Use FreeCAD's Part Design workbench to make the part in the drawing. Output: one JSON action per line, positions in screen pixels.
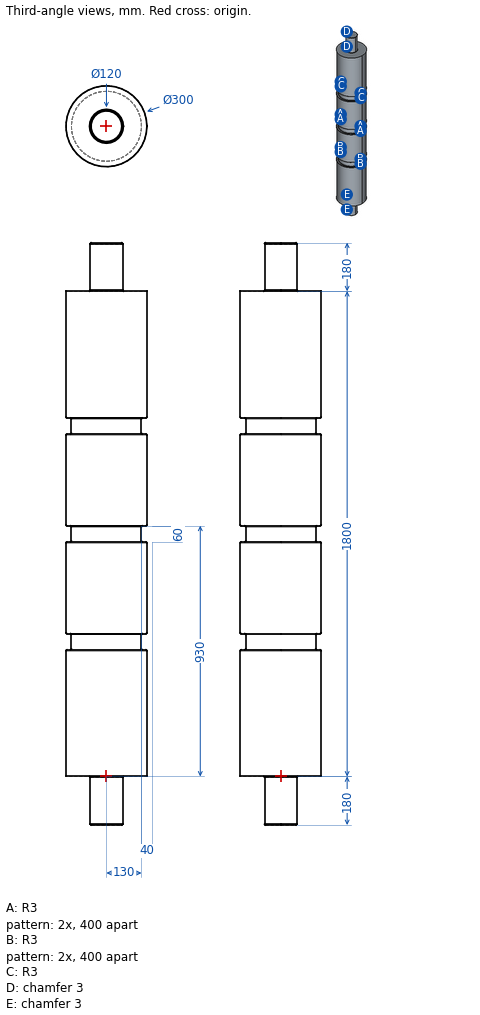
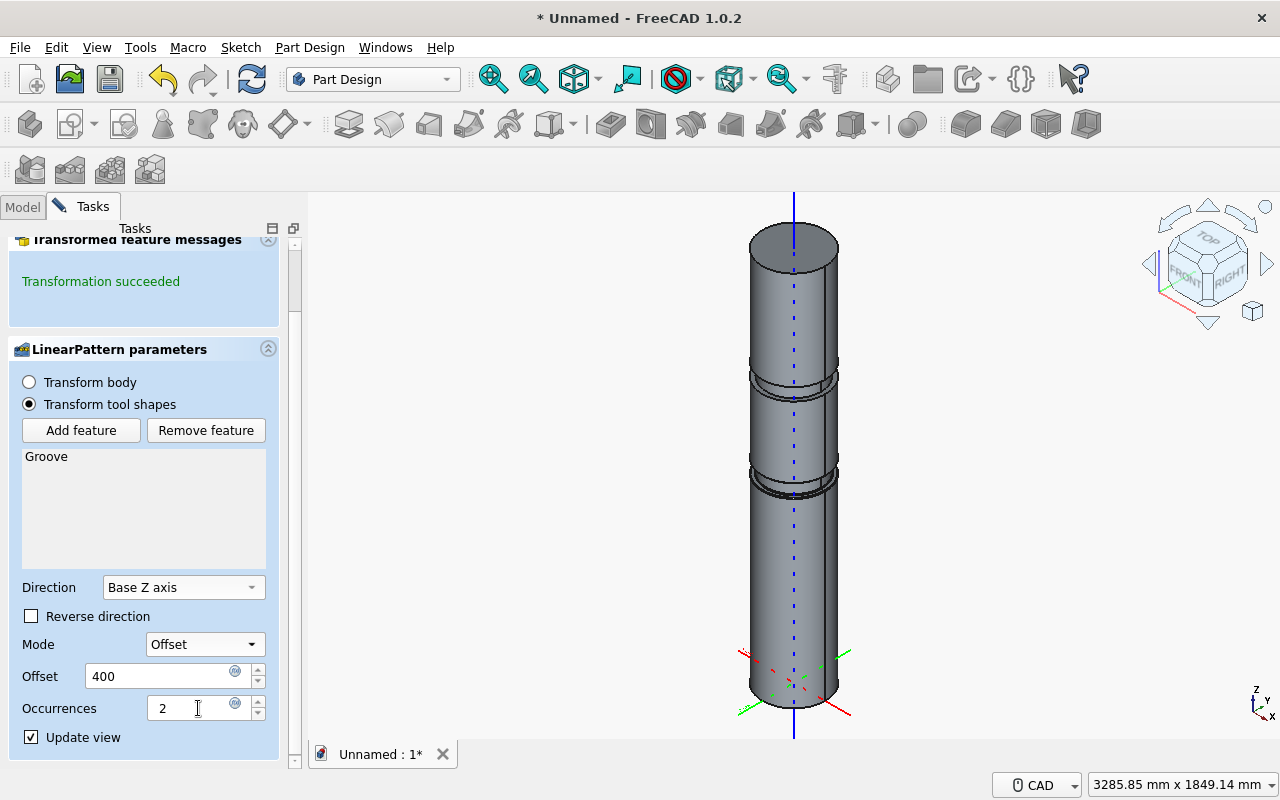
{"action": "left_click", "coordinate": [30, 616]}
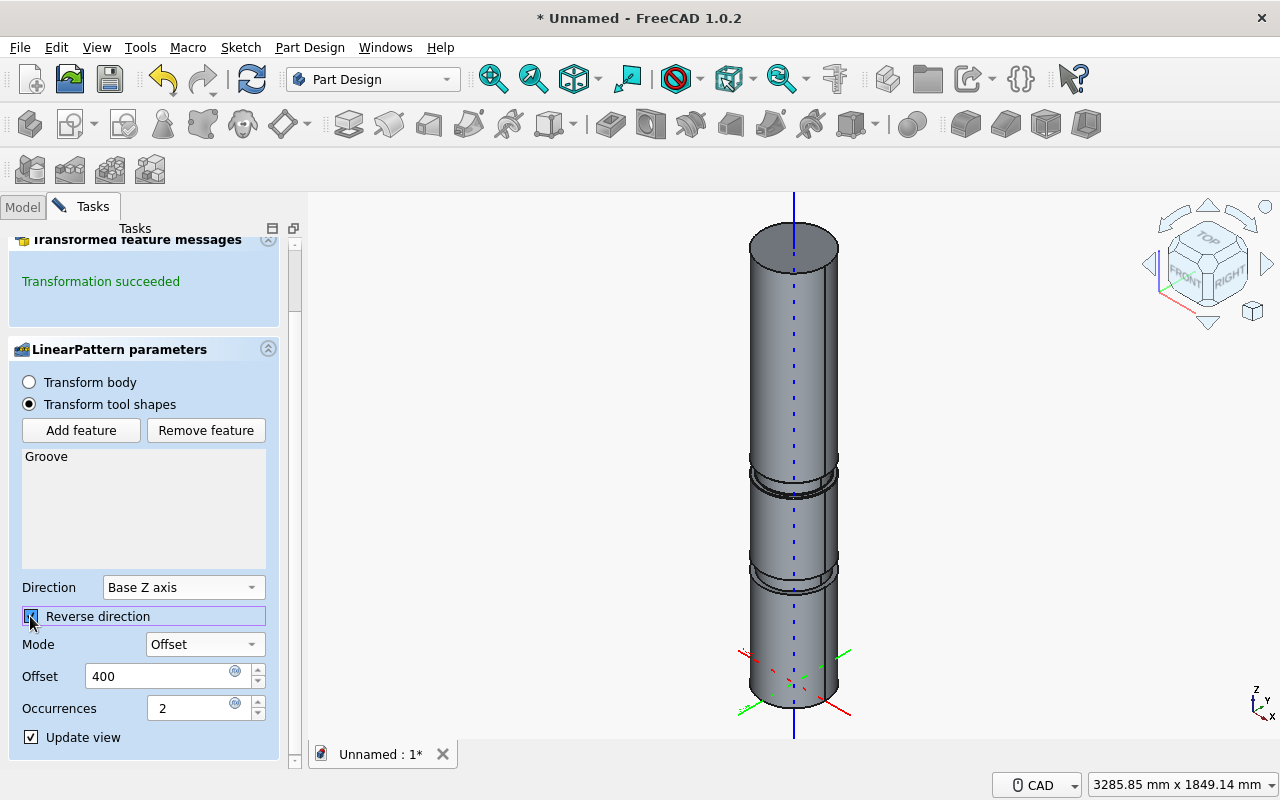
{"action": "scroll", "coordinate": [295, 503], "scroll_direction": "up", "scroll_amount": 2}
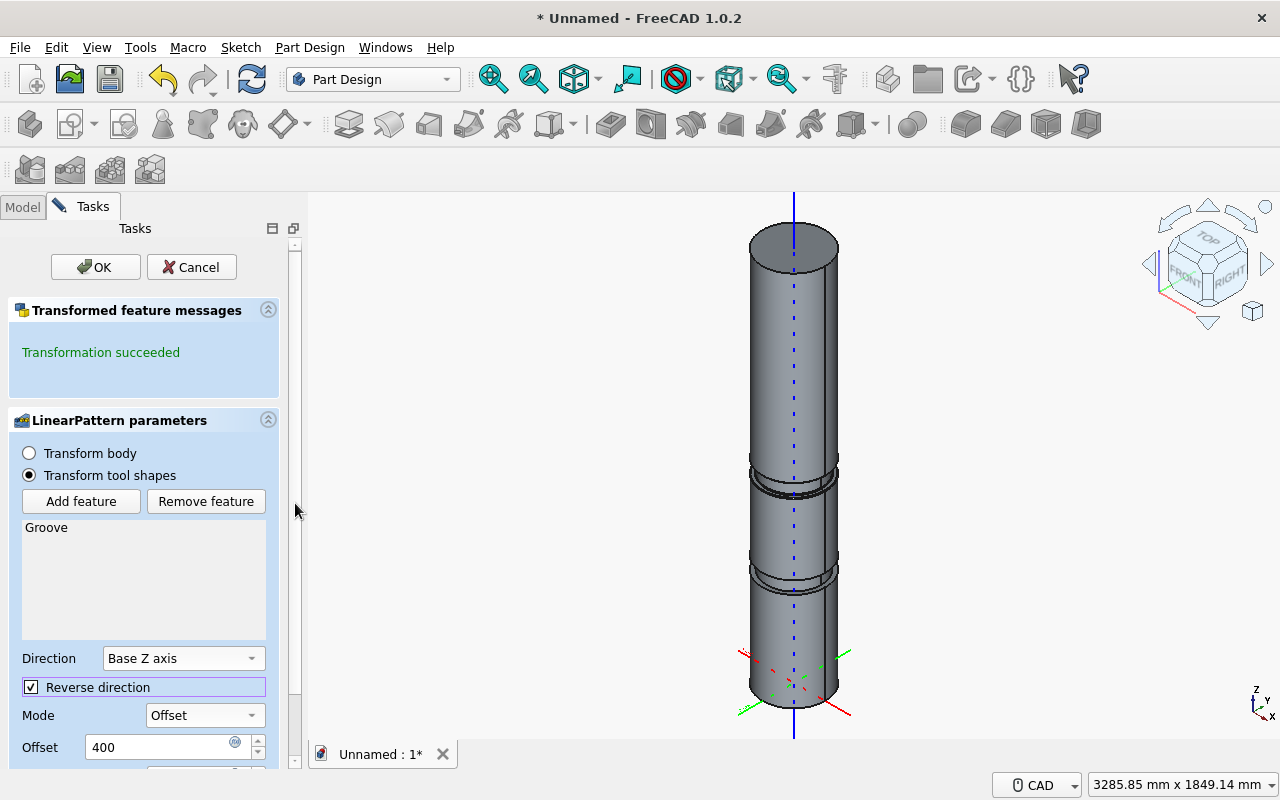
{"action": "left_click", "coordinate": [96, 267]}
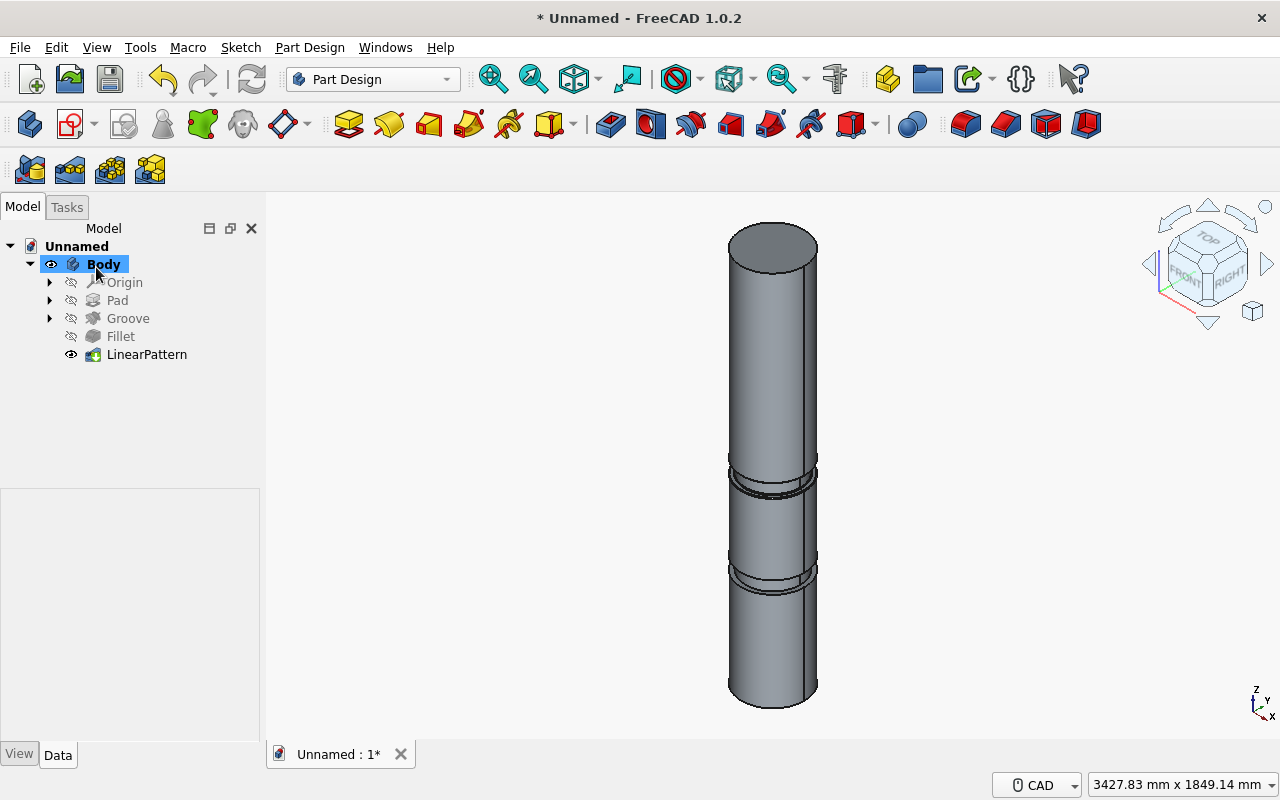
{"action": "left_click", "coordinate": [733, 580]}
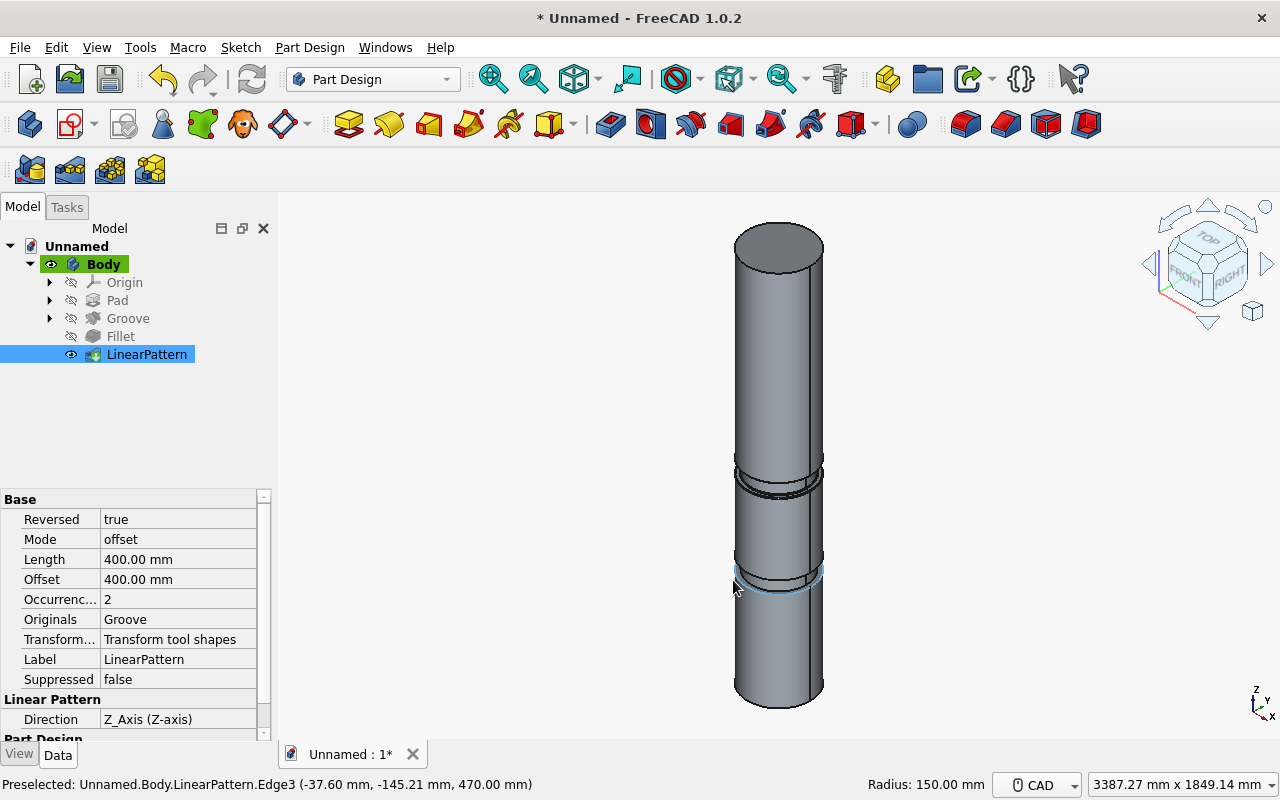
{"action": "key", "text": "2"}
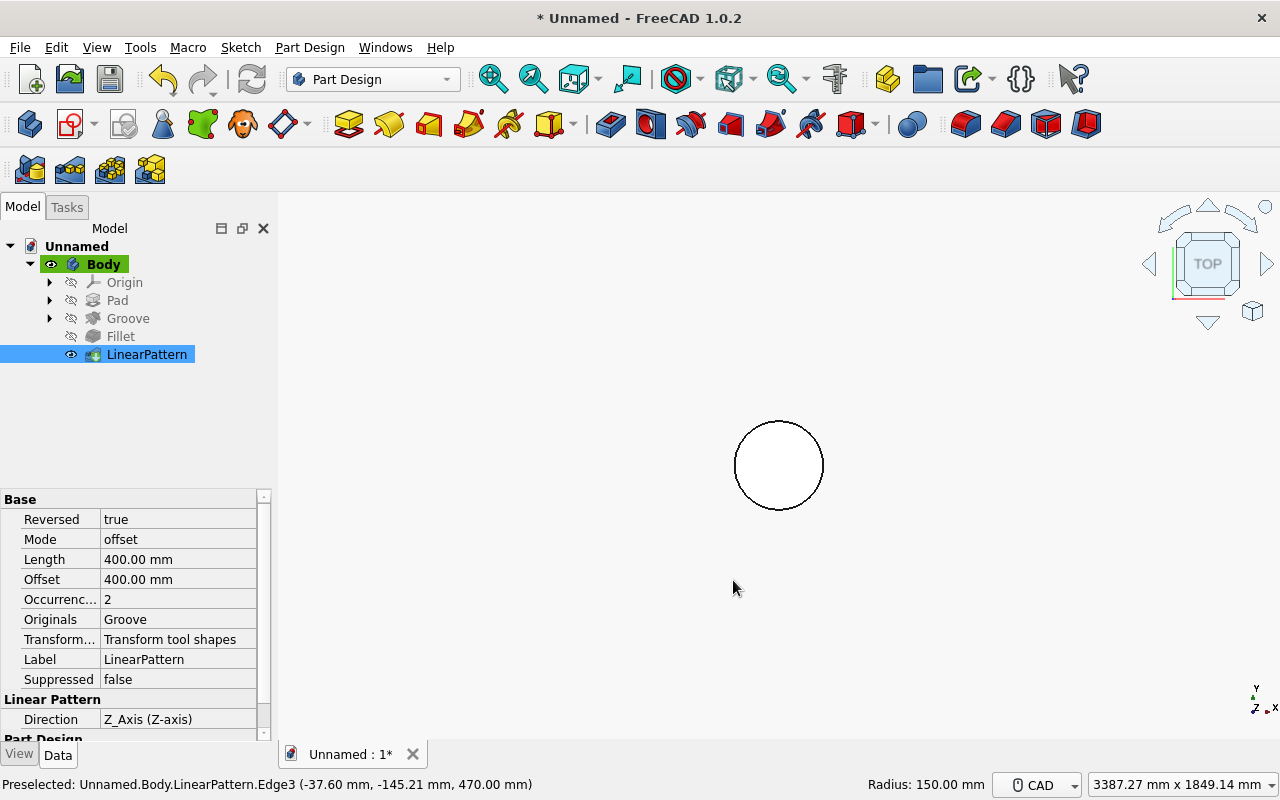
{"action": "key", "text": "v f"}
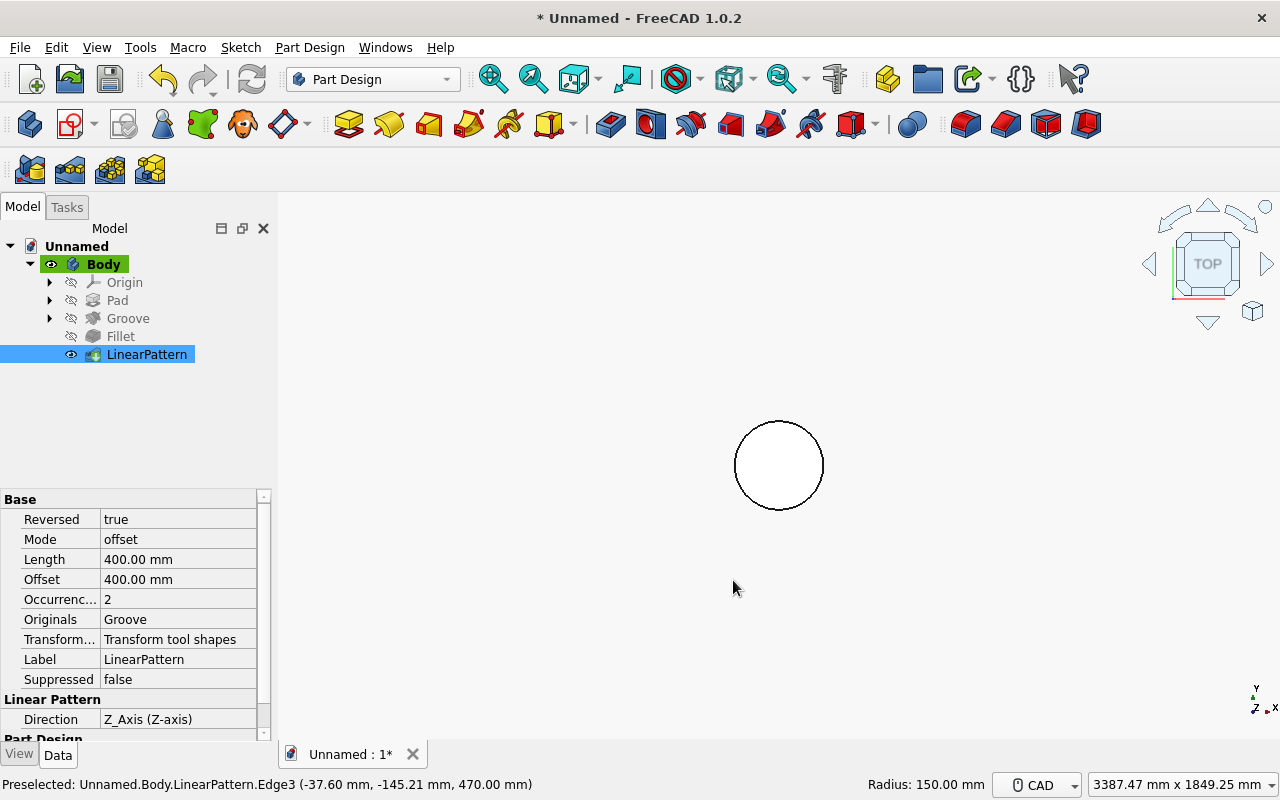
{"action": "key", "text": "0"}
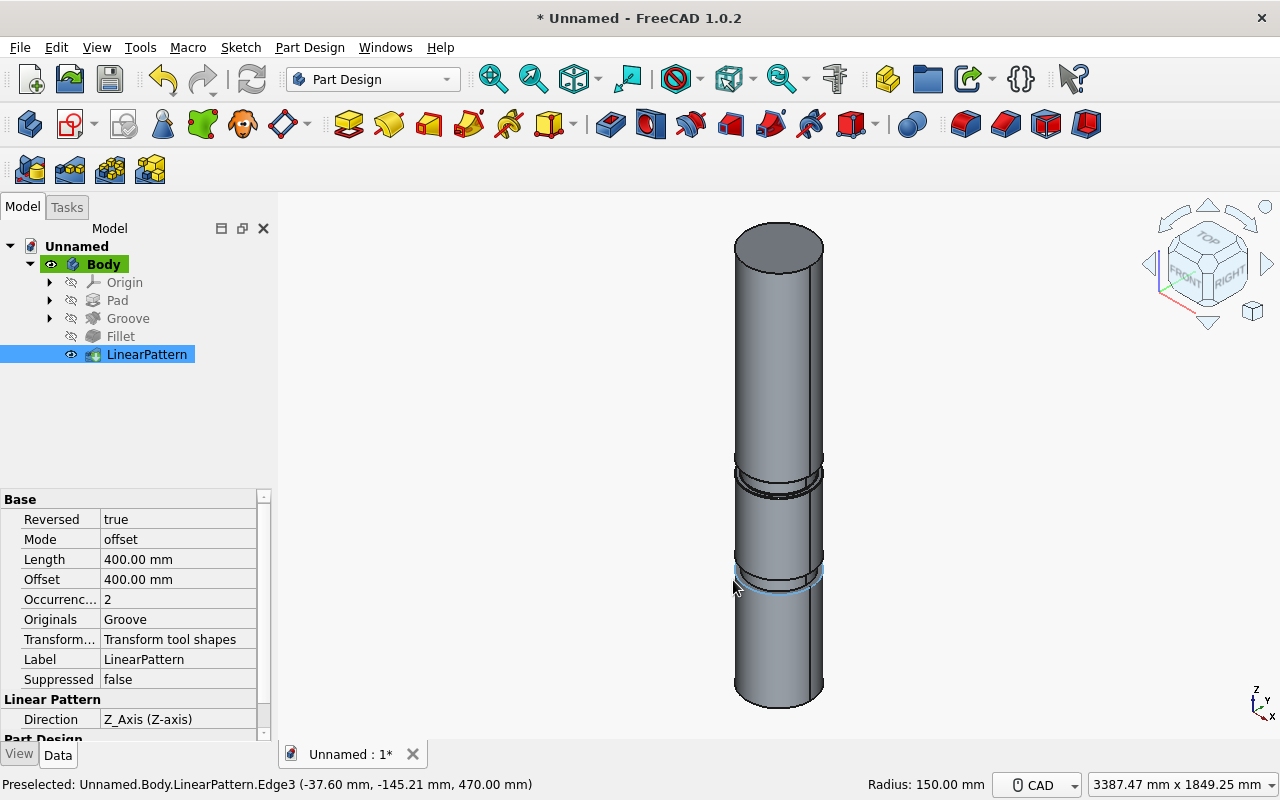
{"action": "key", "text": "1"}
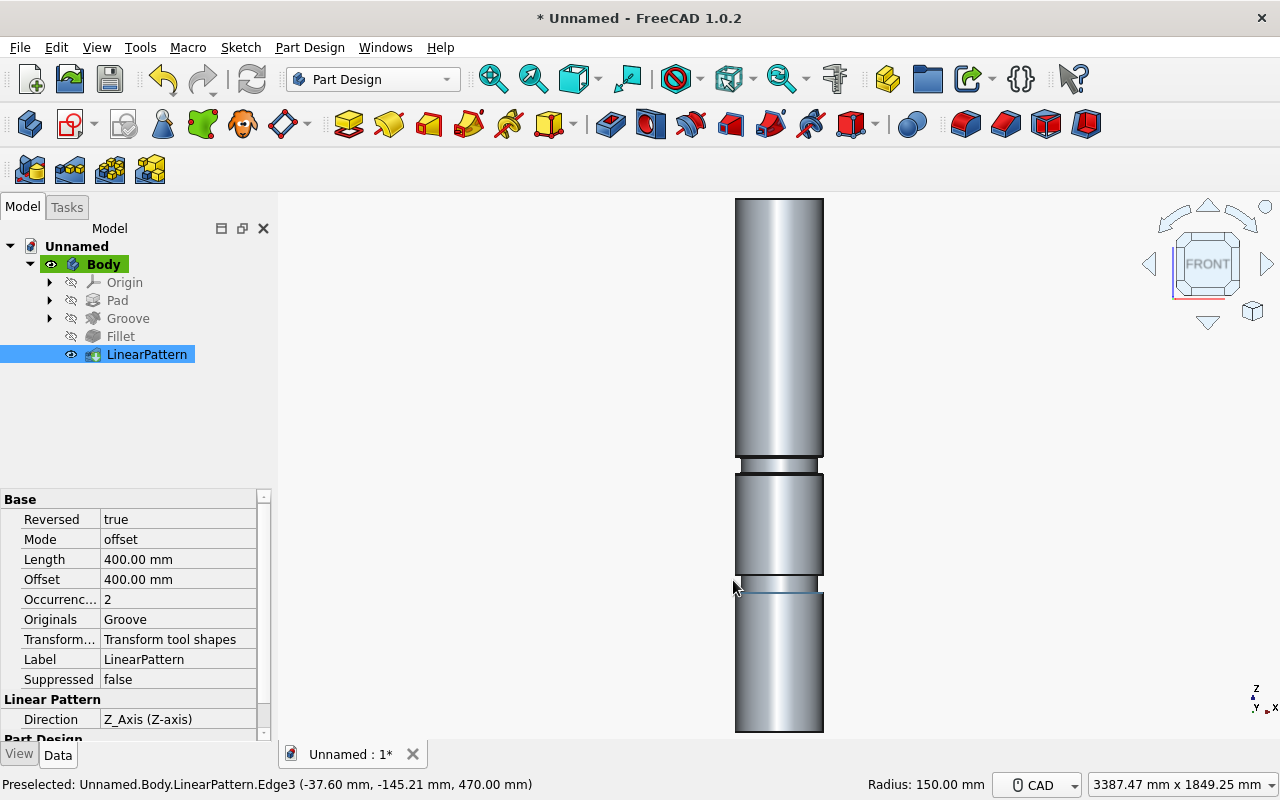
{"action": "left_click", "coordinate": [735, 574], "text": "ctrl"}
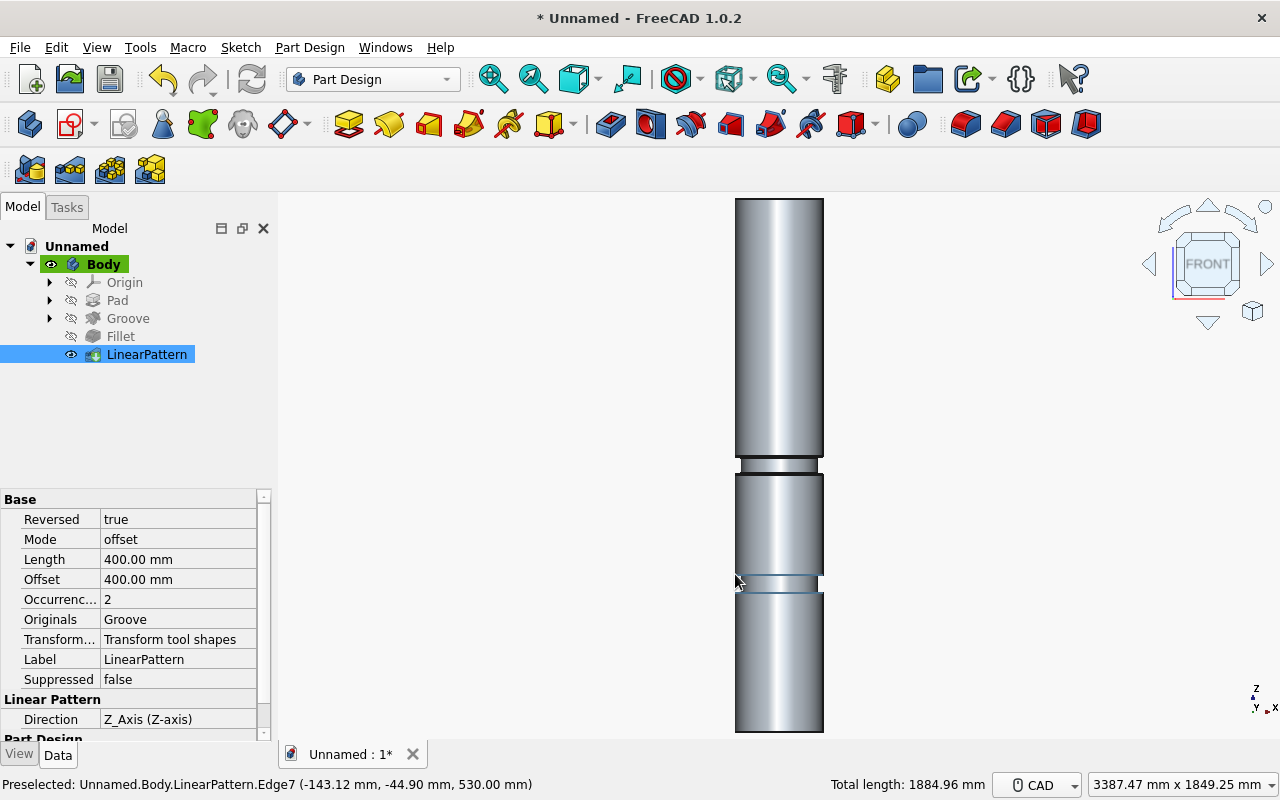
{"action": "key", "text": "3"}